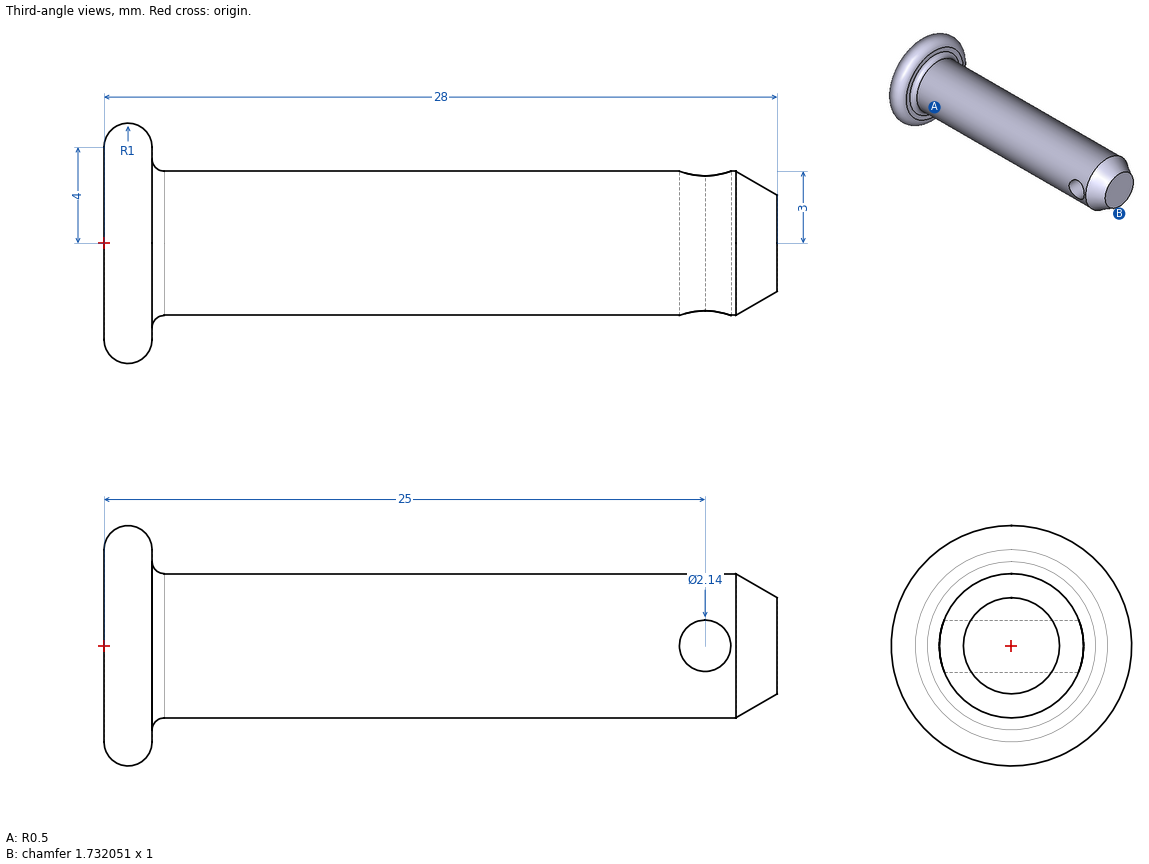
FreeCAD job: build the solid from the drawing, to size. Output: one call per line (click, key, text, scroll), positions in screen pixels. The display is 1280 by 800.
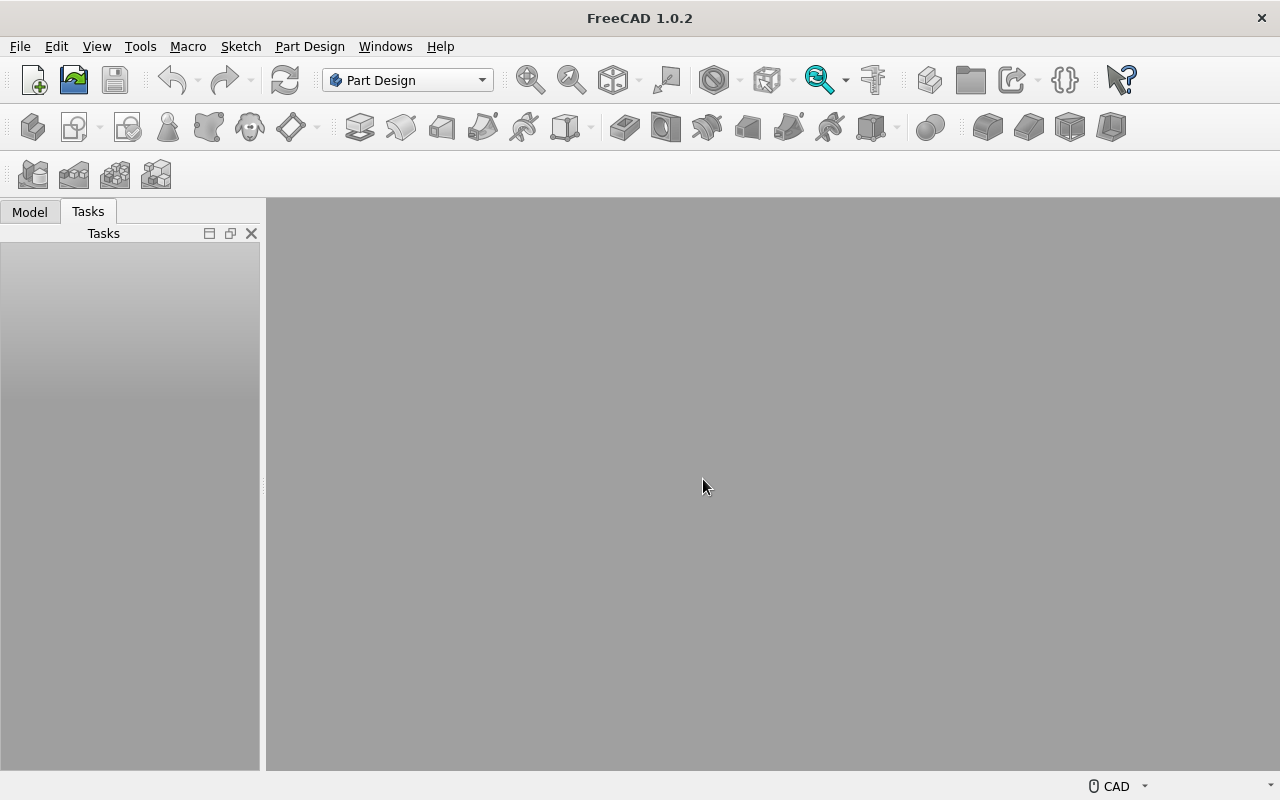
click(33, 80)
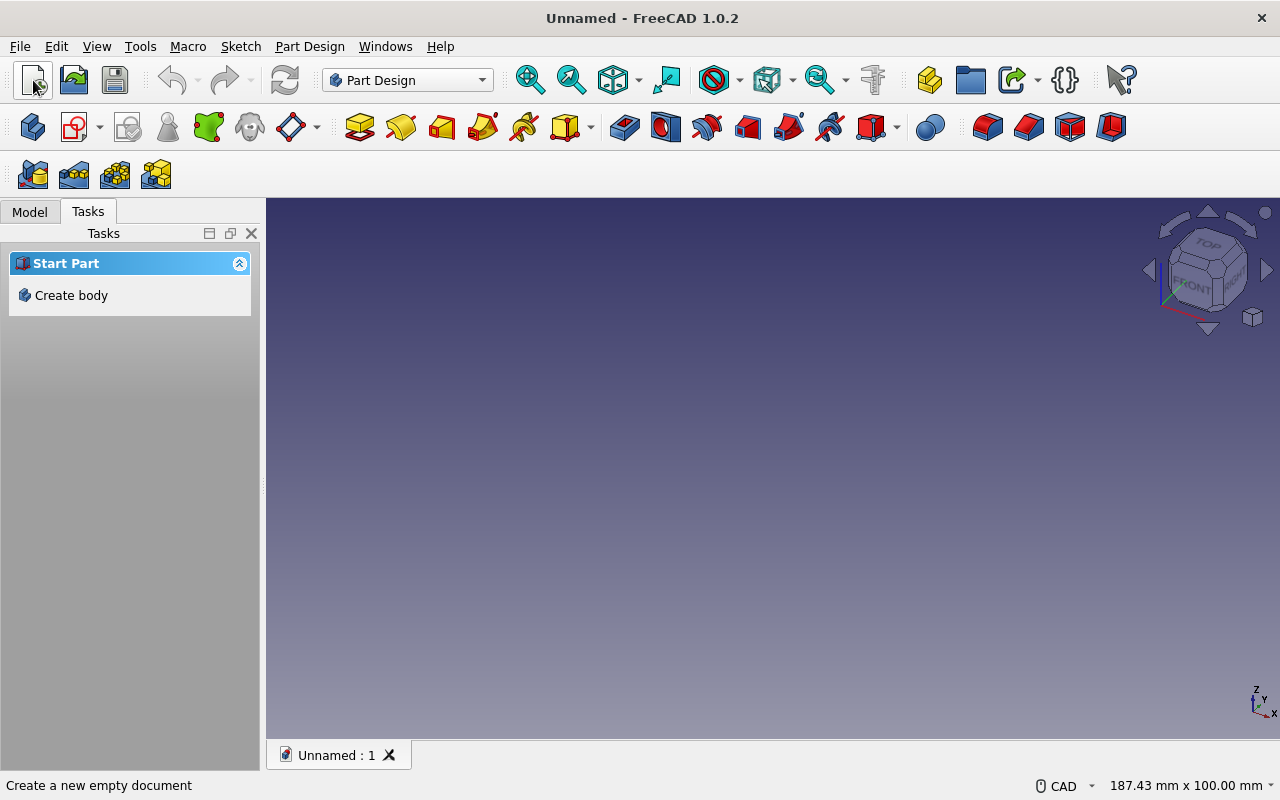
click(74, 128)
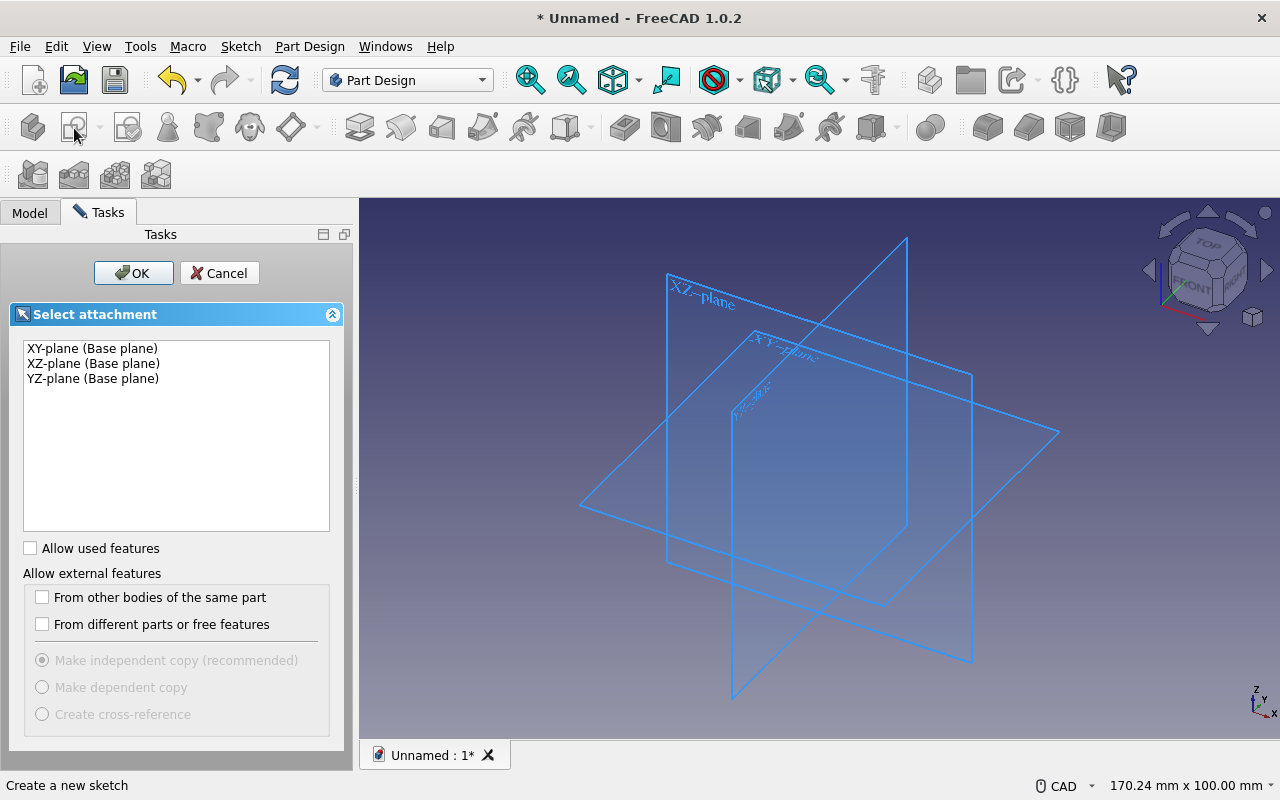
click(84, 348)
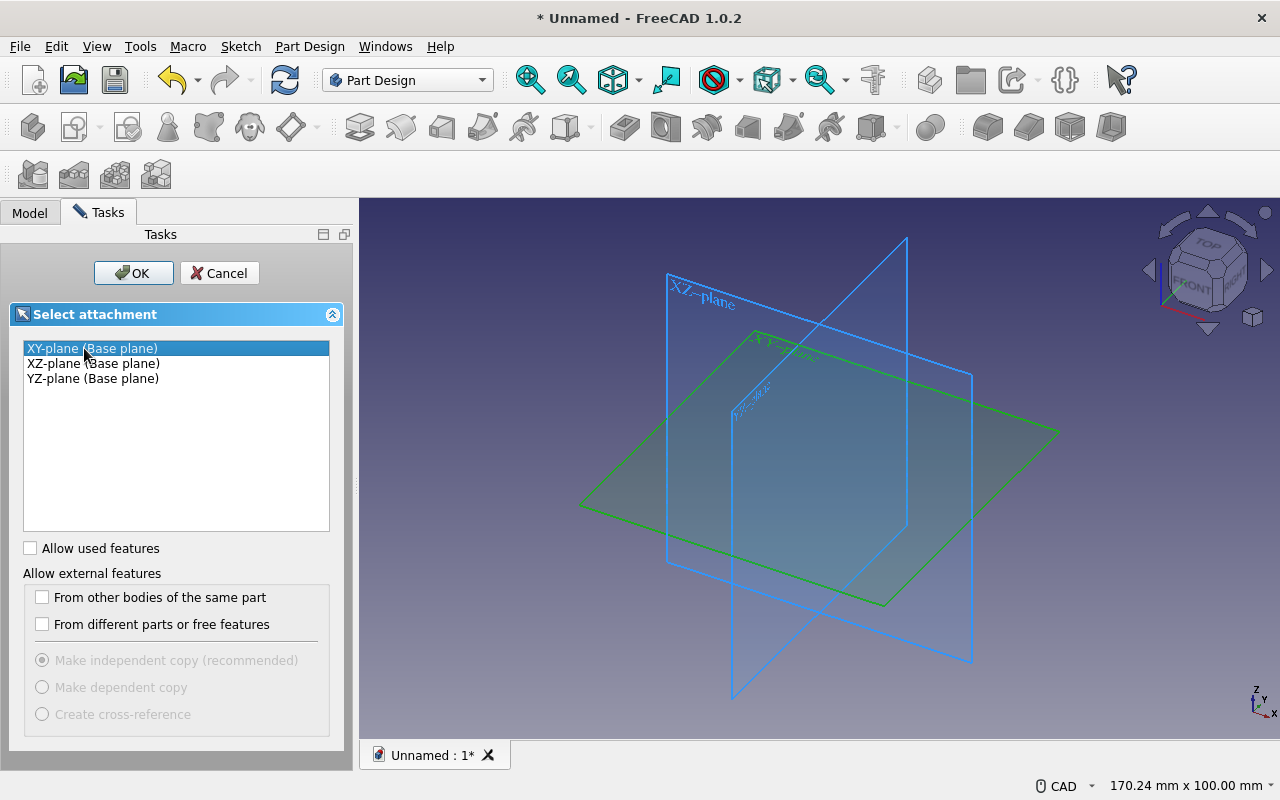
click(134, 273)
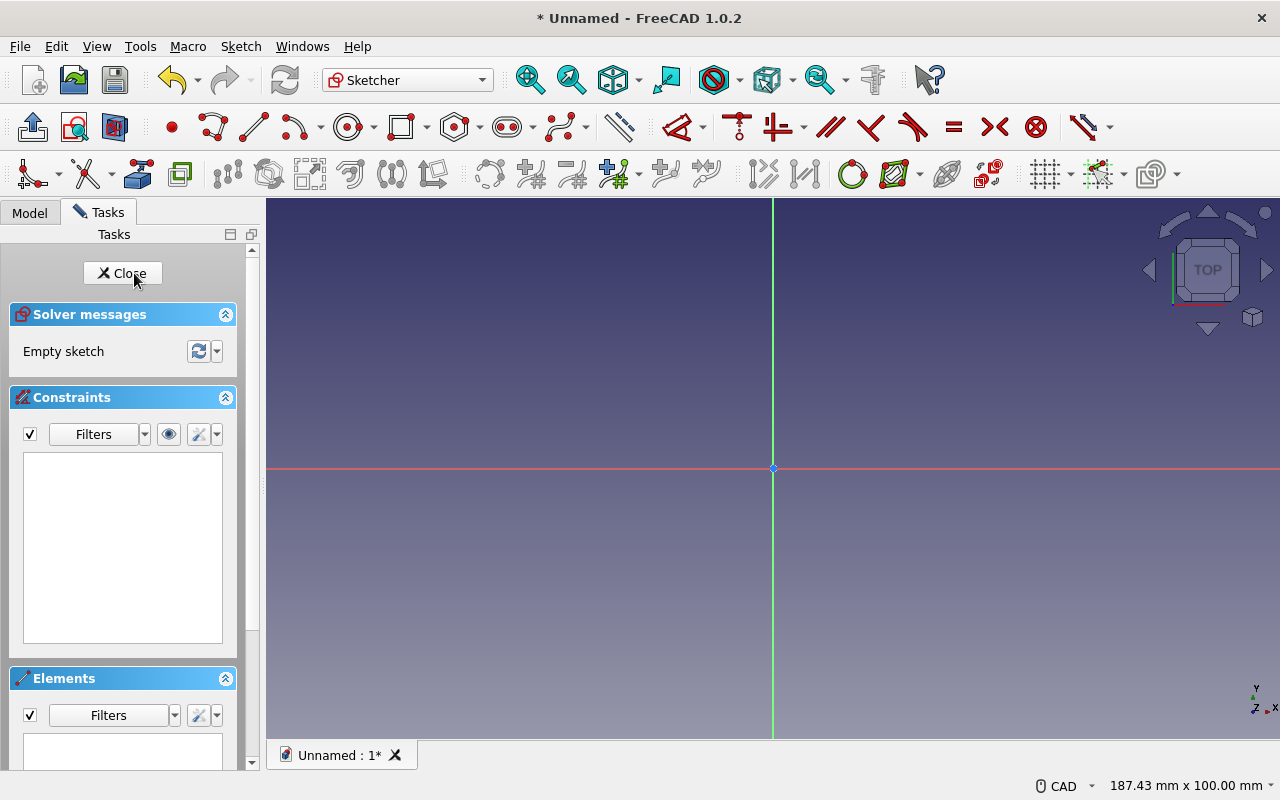
scroll(896, 451, up, 7)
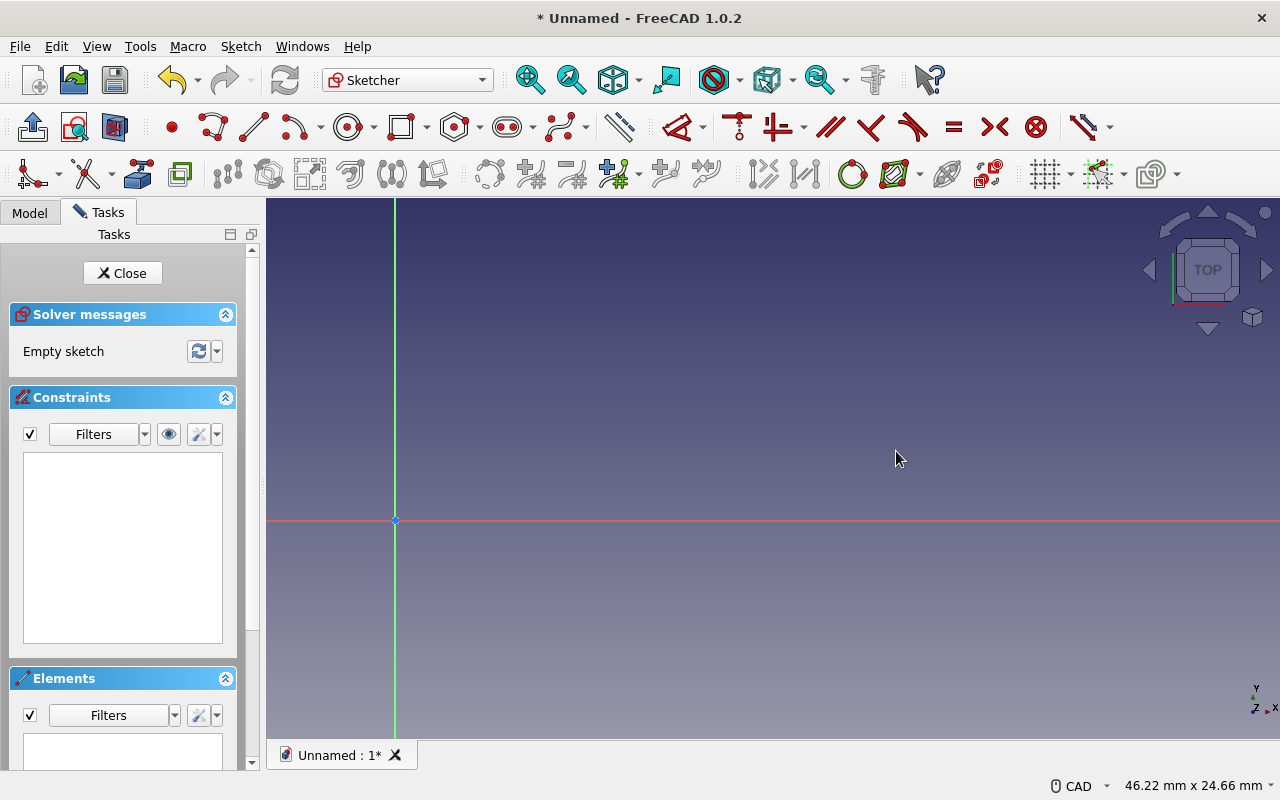
key(g)
key(m)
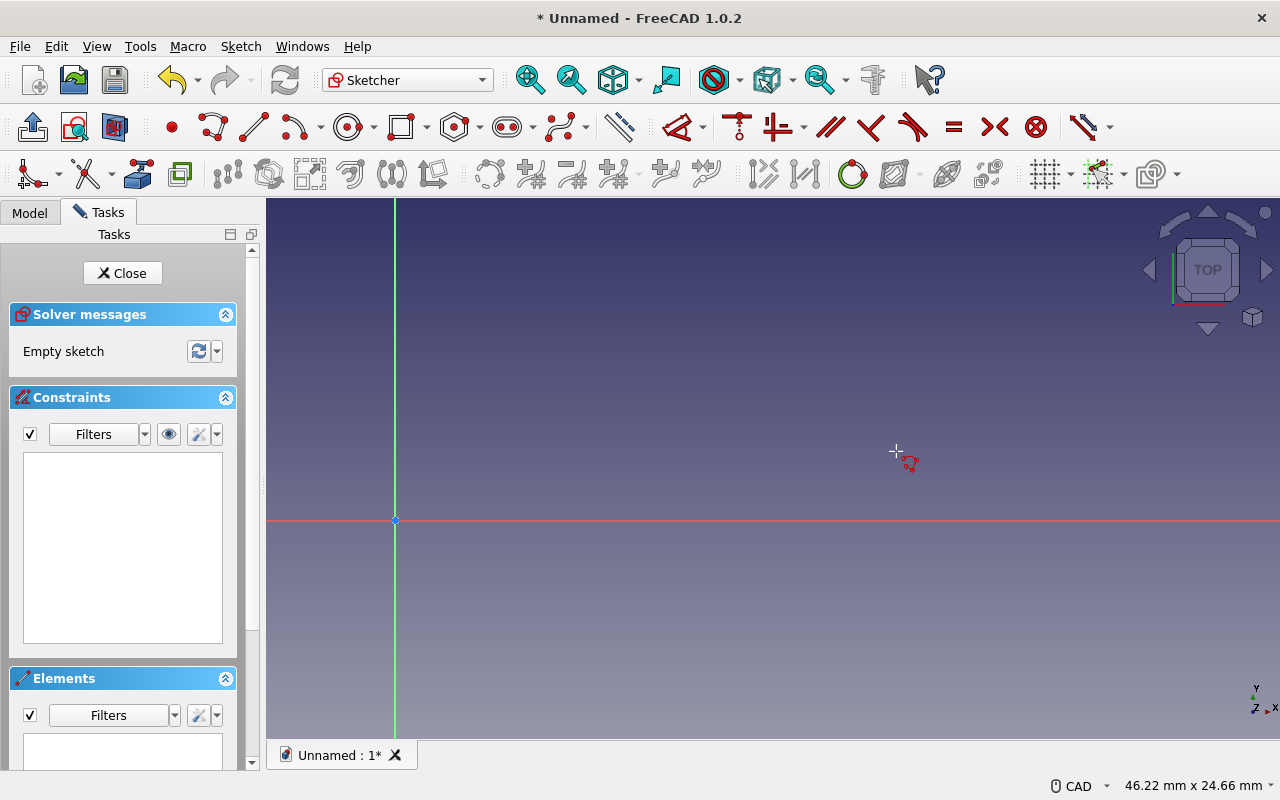
click(395, 433)
click(395, 521)
click(1010, 512)
click(1010, 455)
click(439, 455)
click(439, 433)
right_click(439, 433)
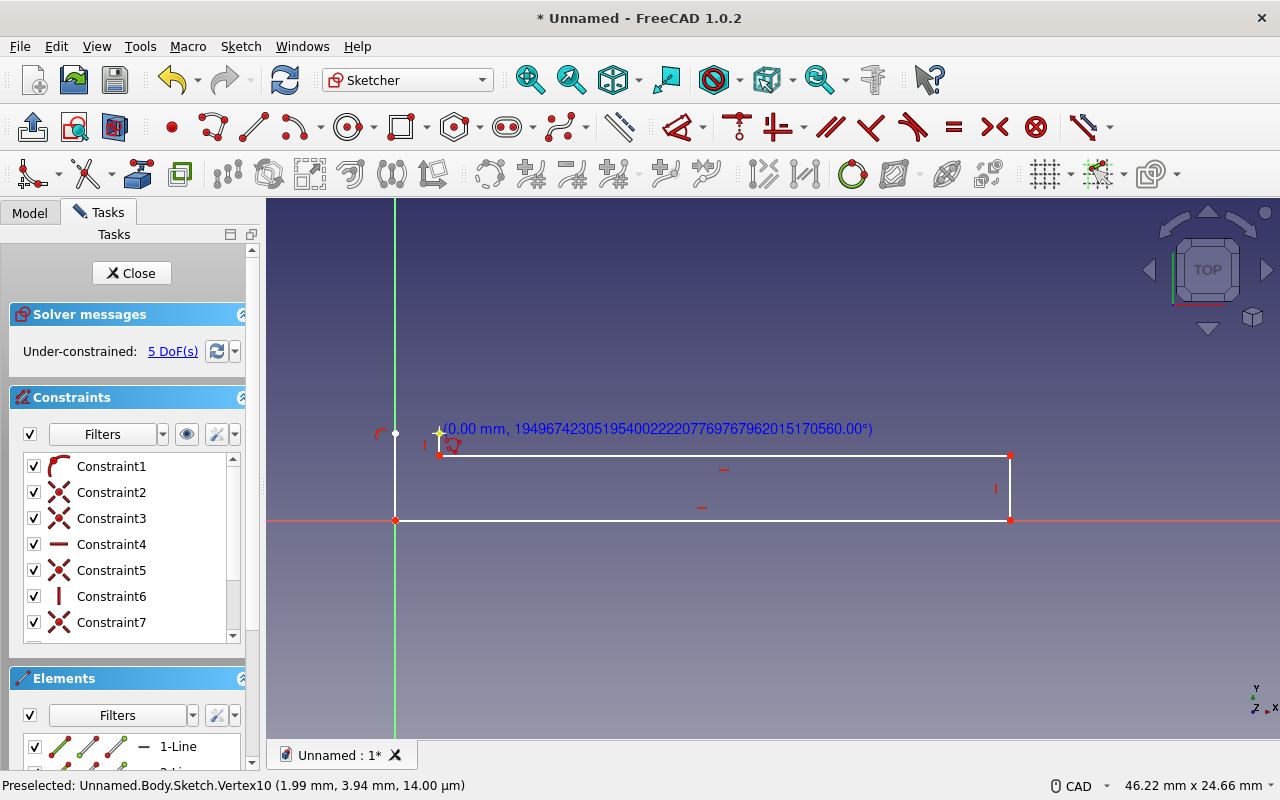
click(320, 128)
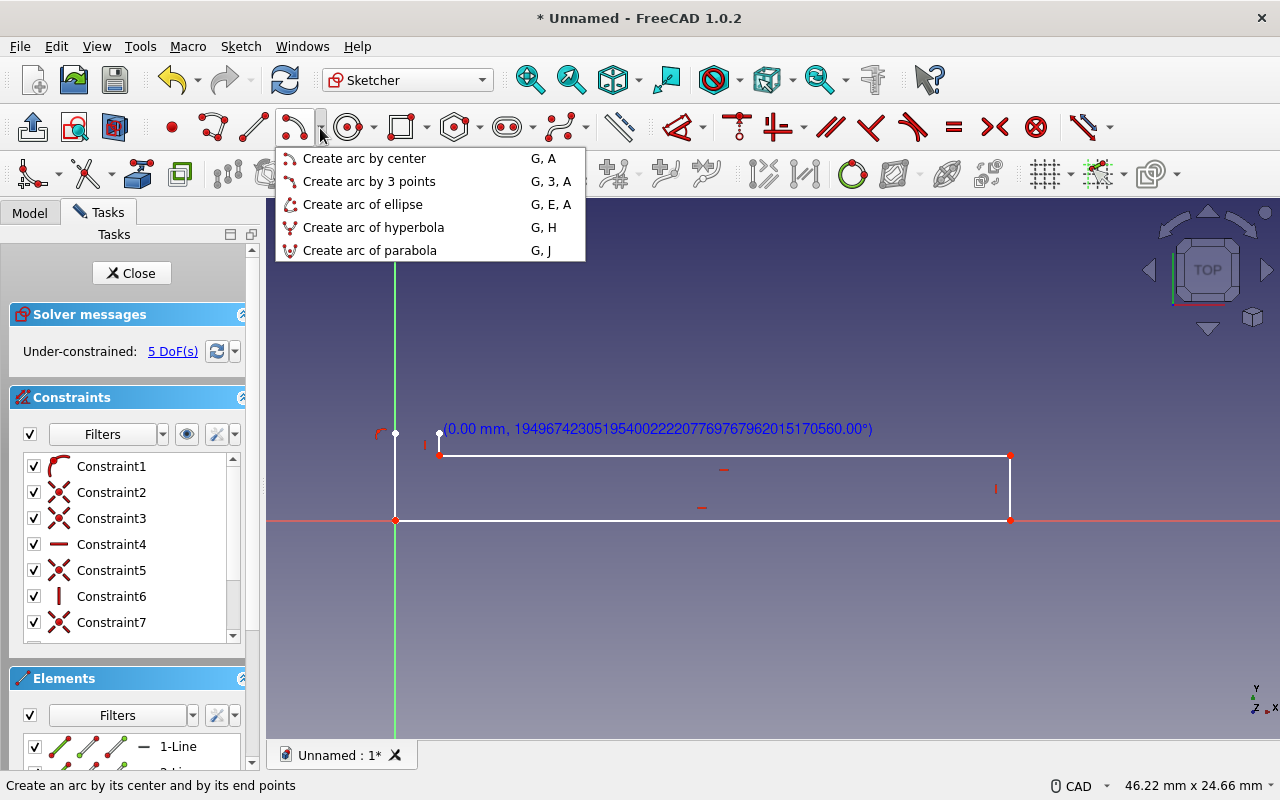
click(430, 182)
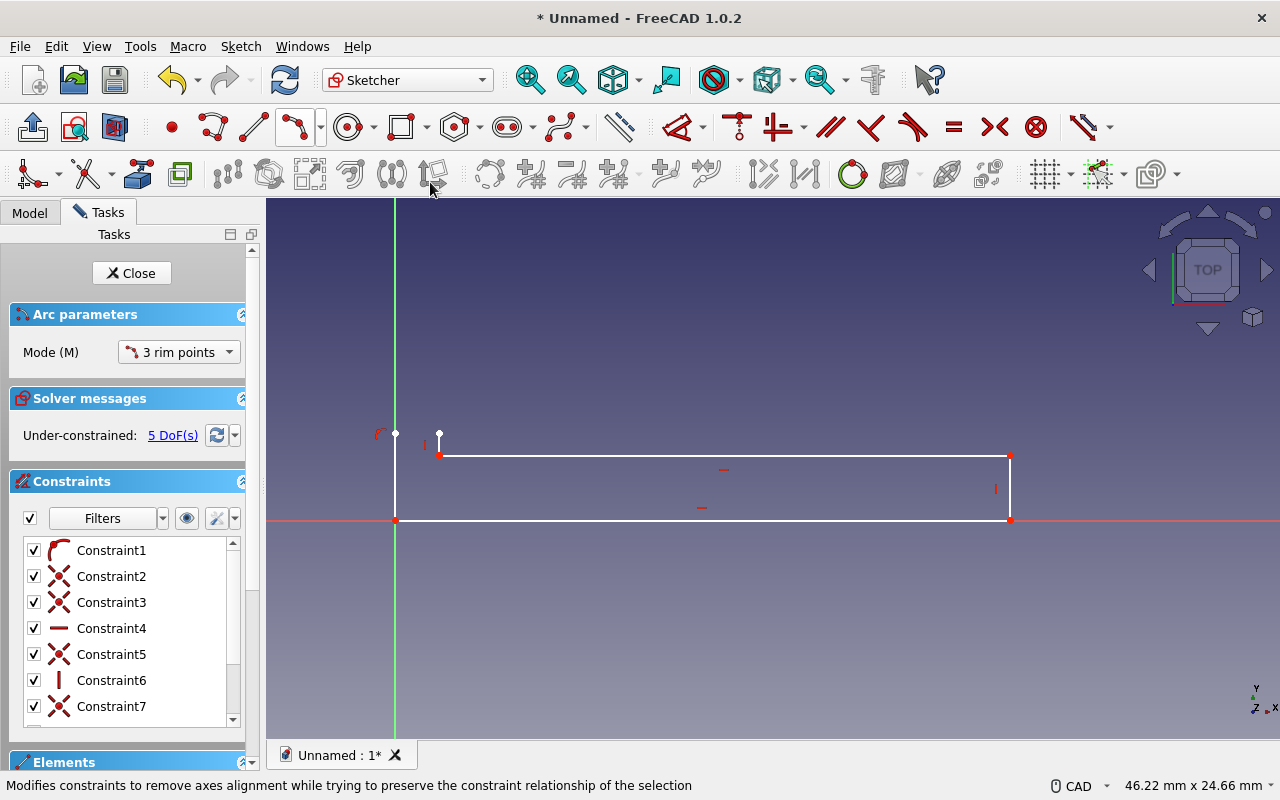
scroll(439, 433, up, 2)